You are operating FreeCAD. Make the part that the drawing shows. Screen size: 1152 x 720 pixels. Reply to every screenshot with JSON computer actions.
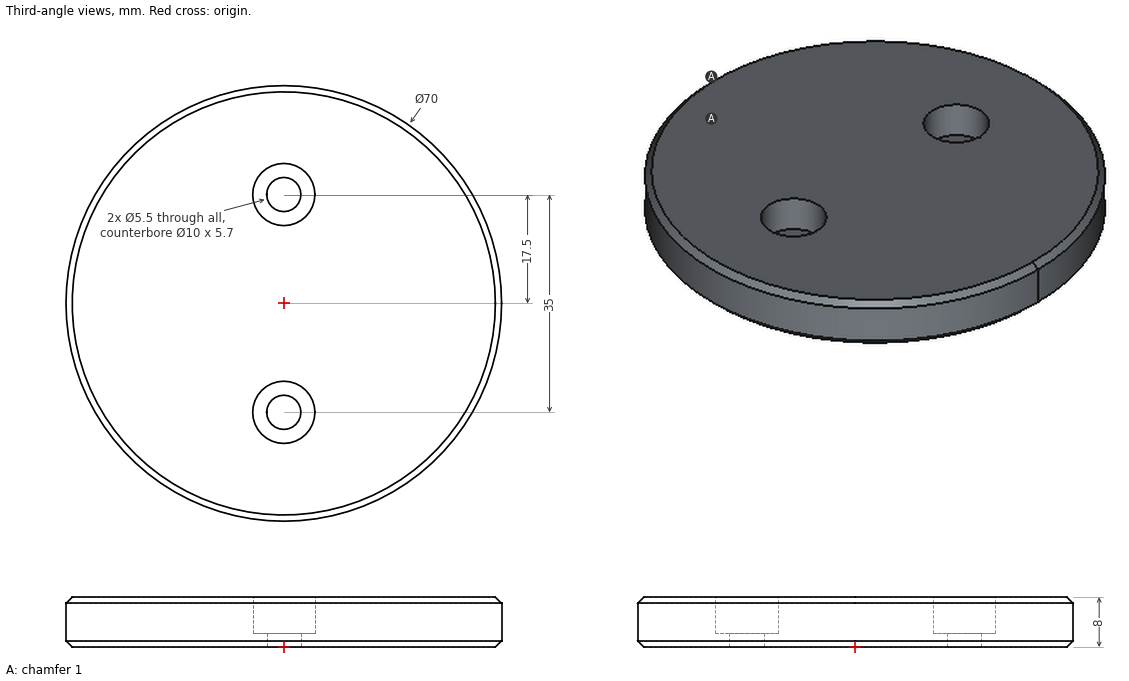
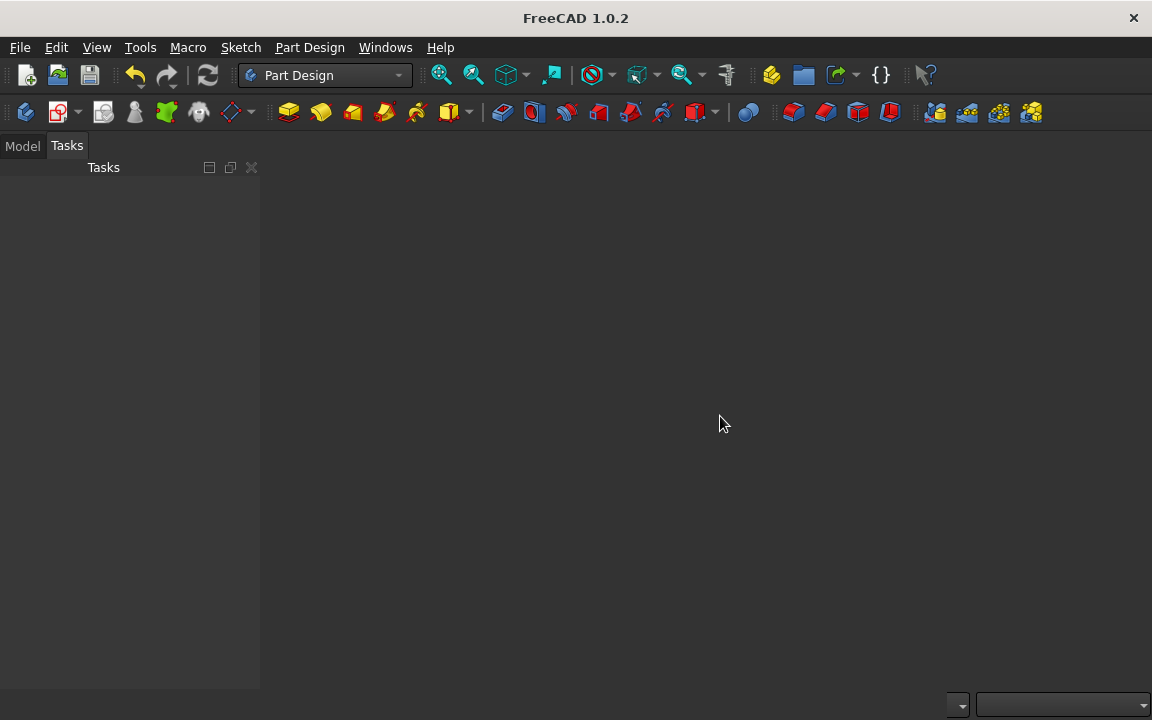
{"action": "key", "text": "ctrl+n"}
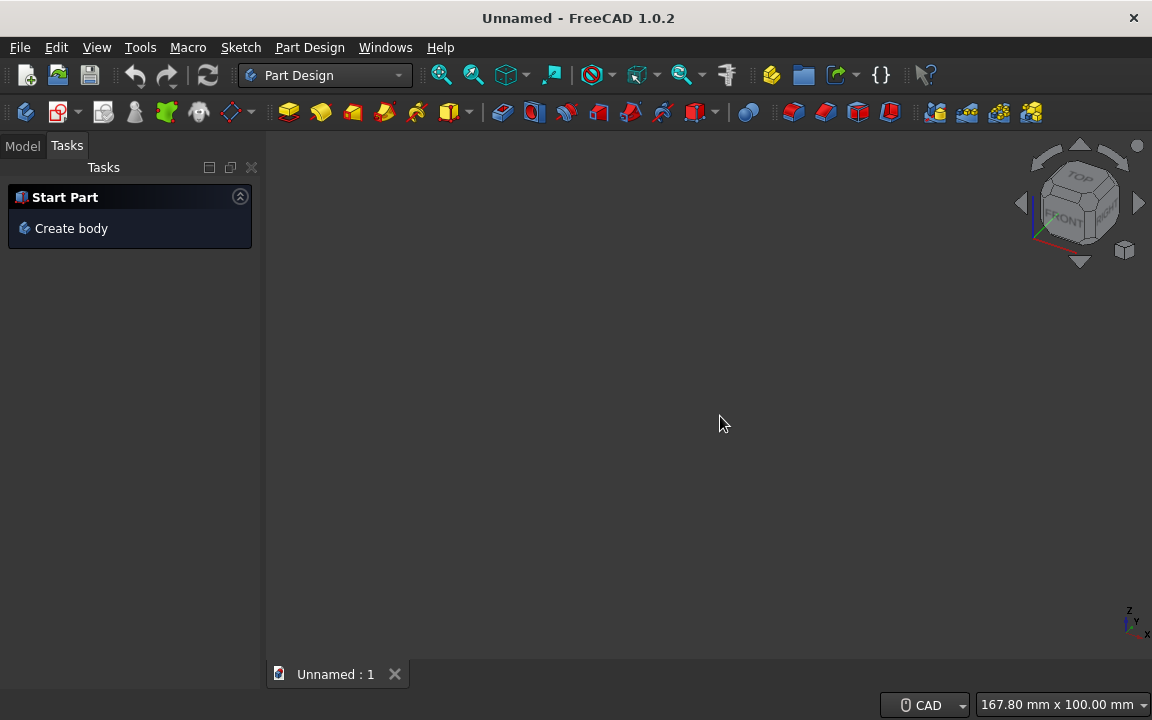
{"action": "left_click", "coordinate": [58, 112]}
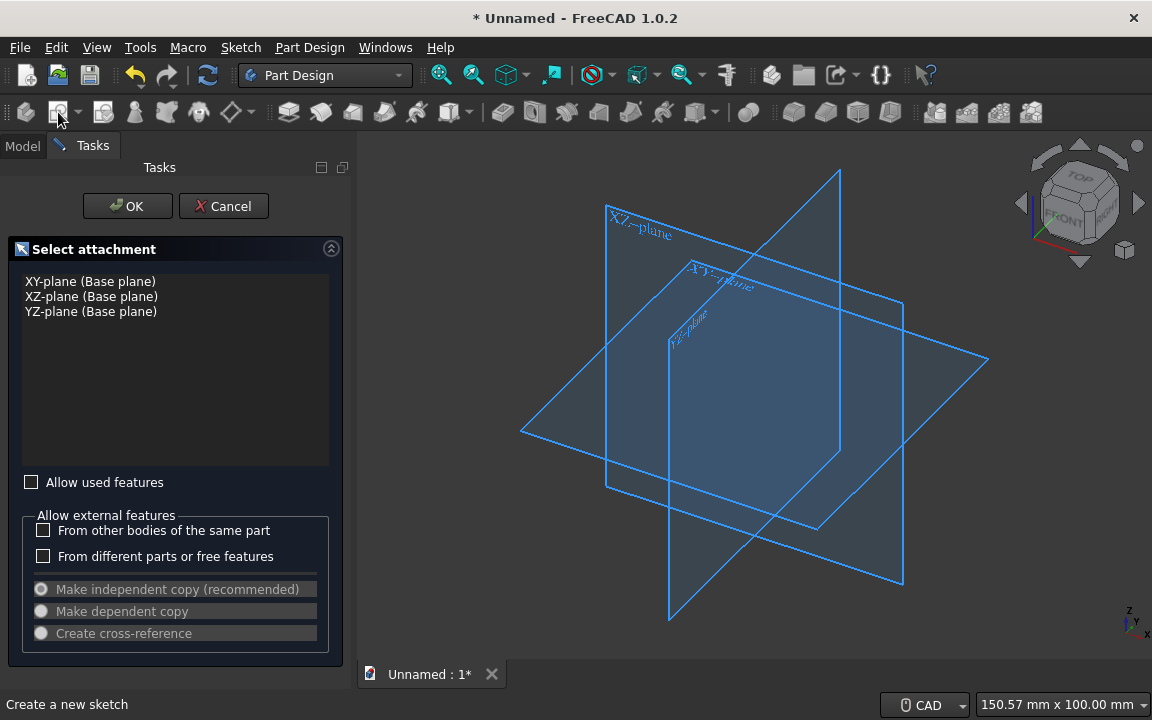
{"action": "left_click", "coordinate": [82, 282]}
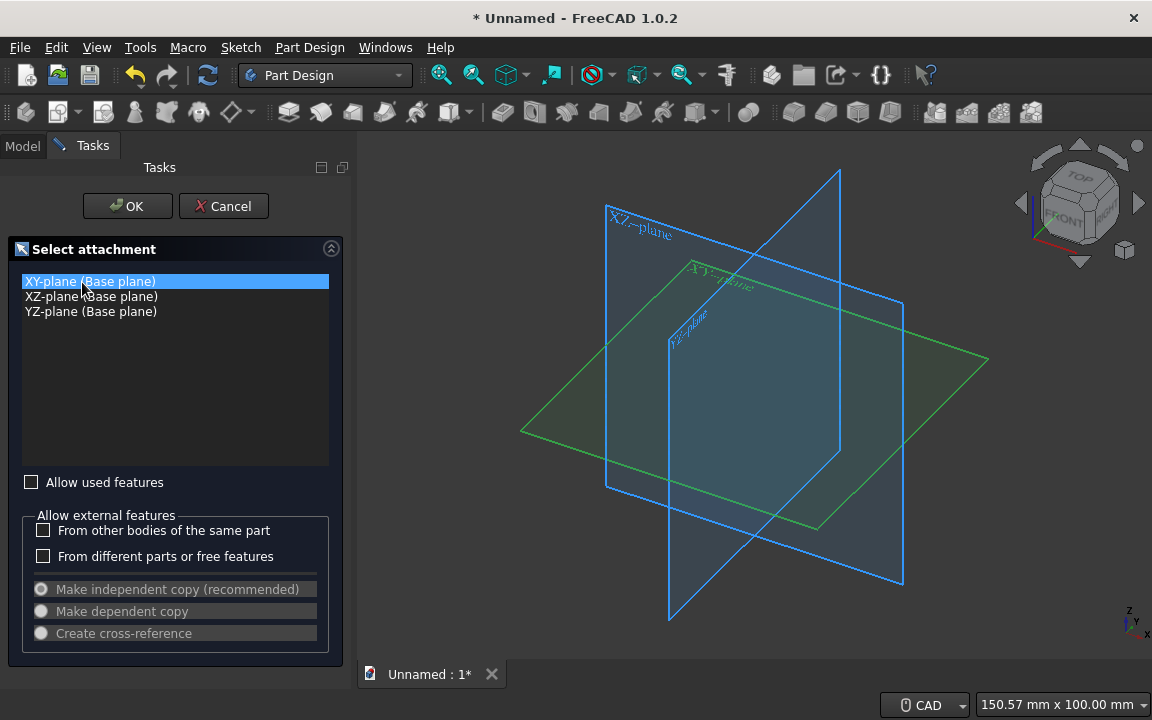
{"action": "left_click", "coordinate": [128, 206]}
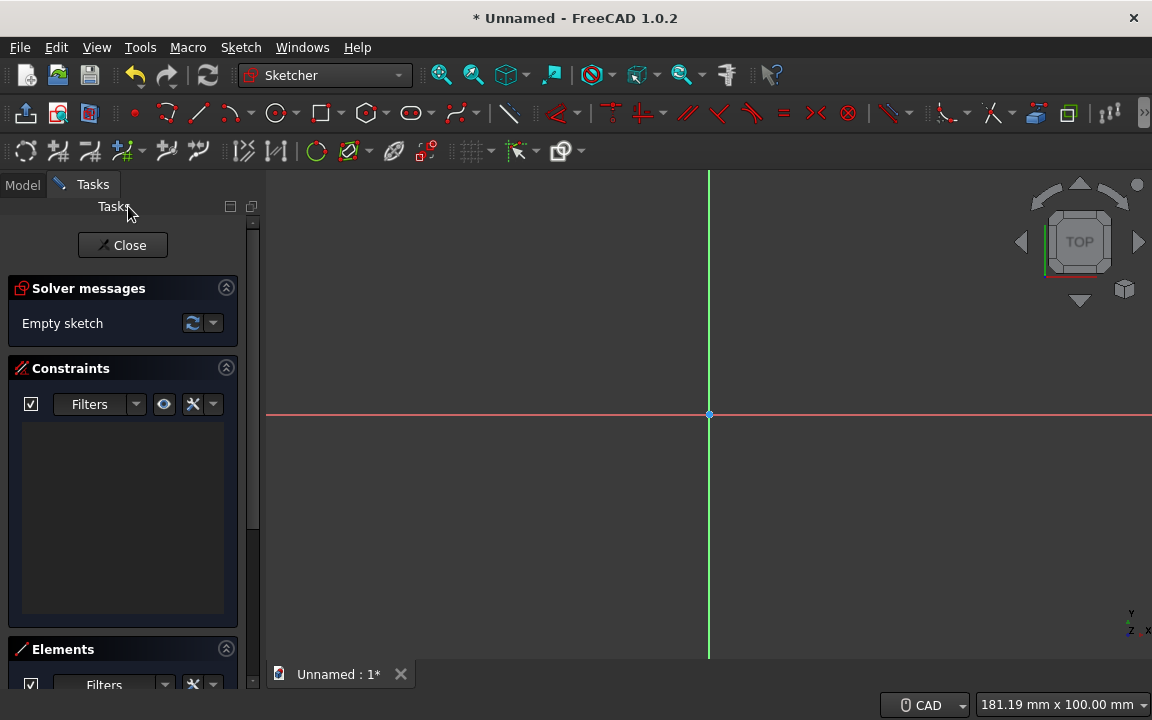
{"action": "left_click", "coordinate": [276, 114]}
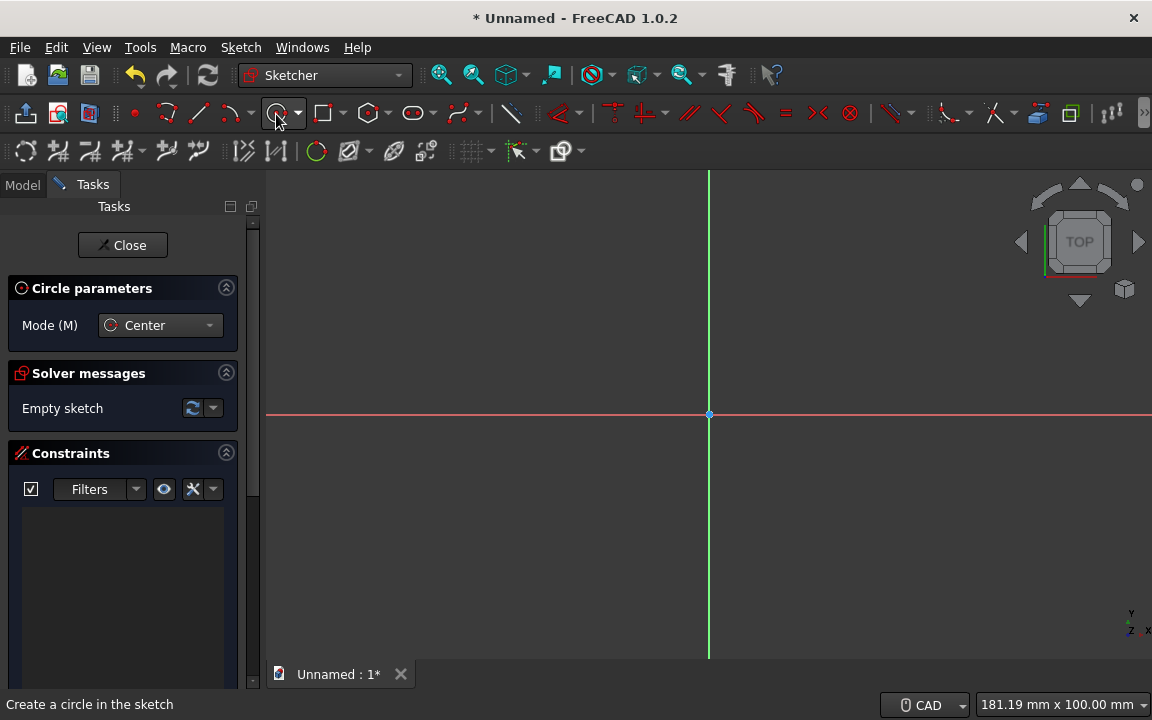
{"action": "left_click", "coordinate": [709, 414]}
{"action": "left_click", "coordinate": [830, 293]}
{"action": "key", "text": "Escape"}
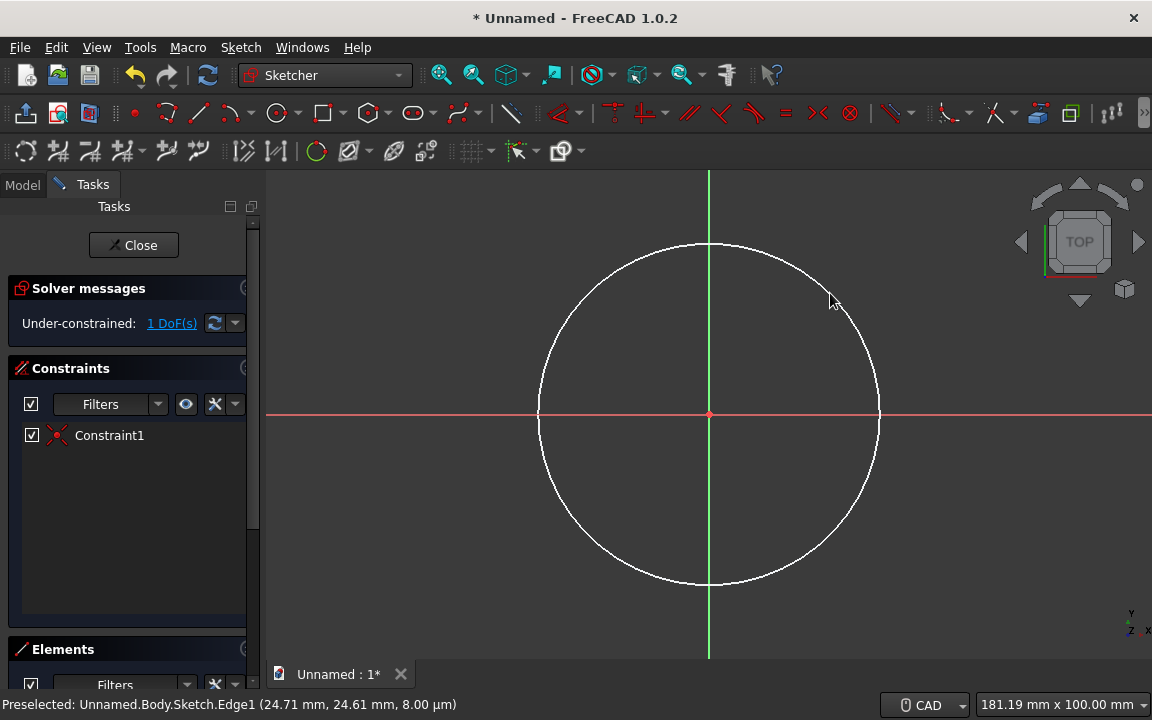
{"action": "left_click", "coordinate": [558, 114]}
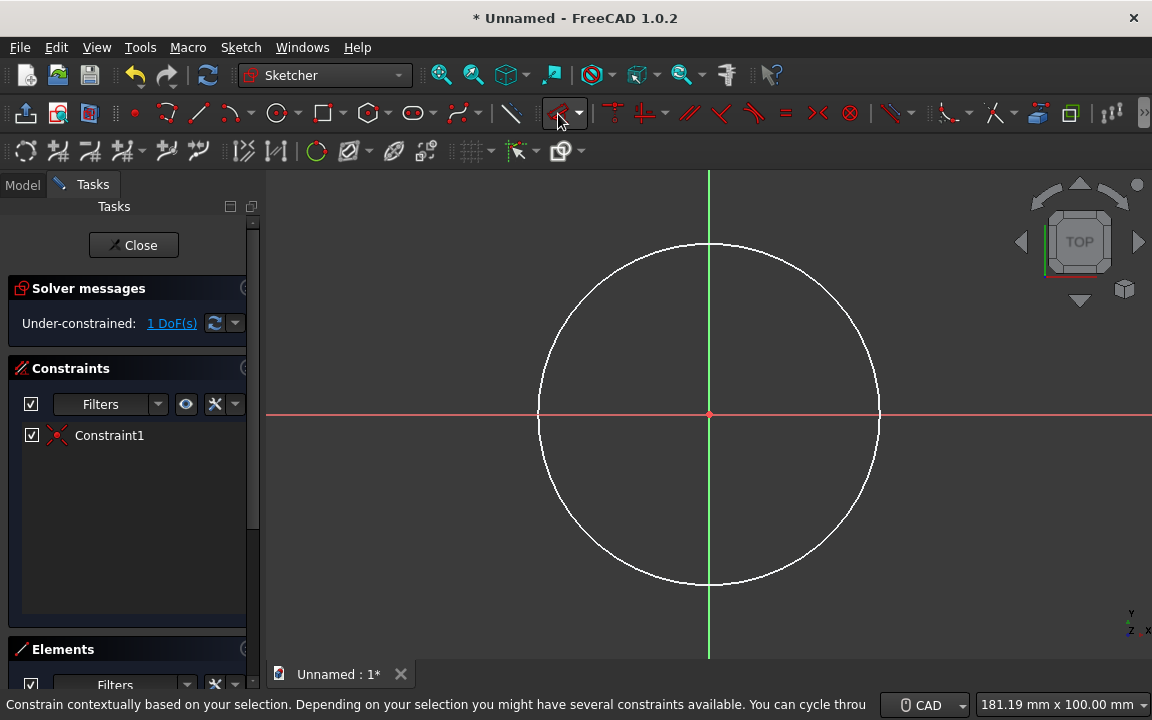
{"action": "left_click", "coordinate": [829, 293]}
{"action": "left_click", "coordinate": [851, 270]}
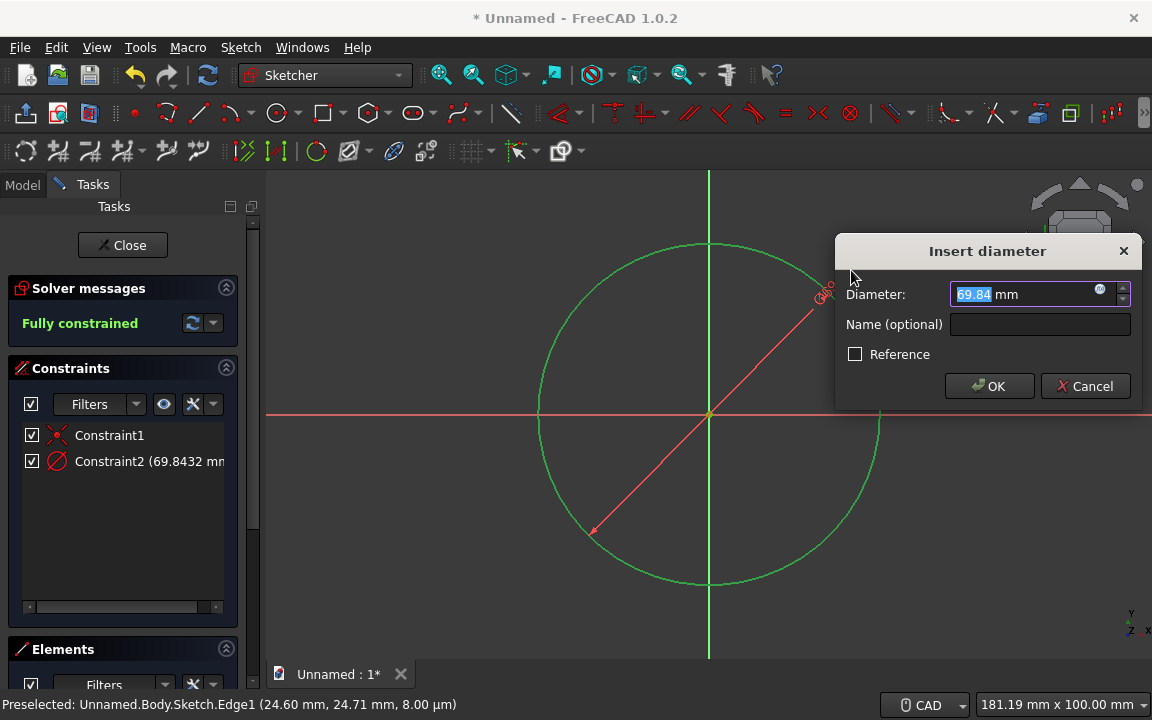
{"action": "type", "text": "70"}
{"action": "key", "text": "Return"}
{"action": "key", "text": "Escape"}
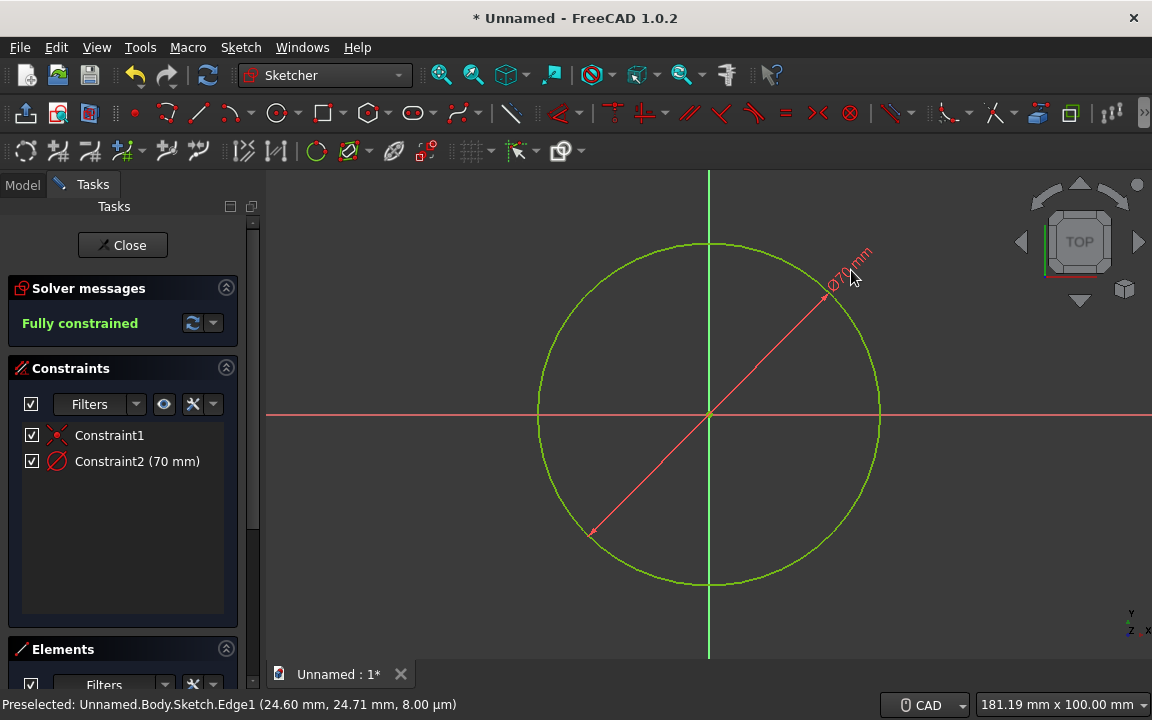
{"action": "left_click", "coordinate": [123, 245]}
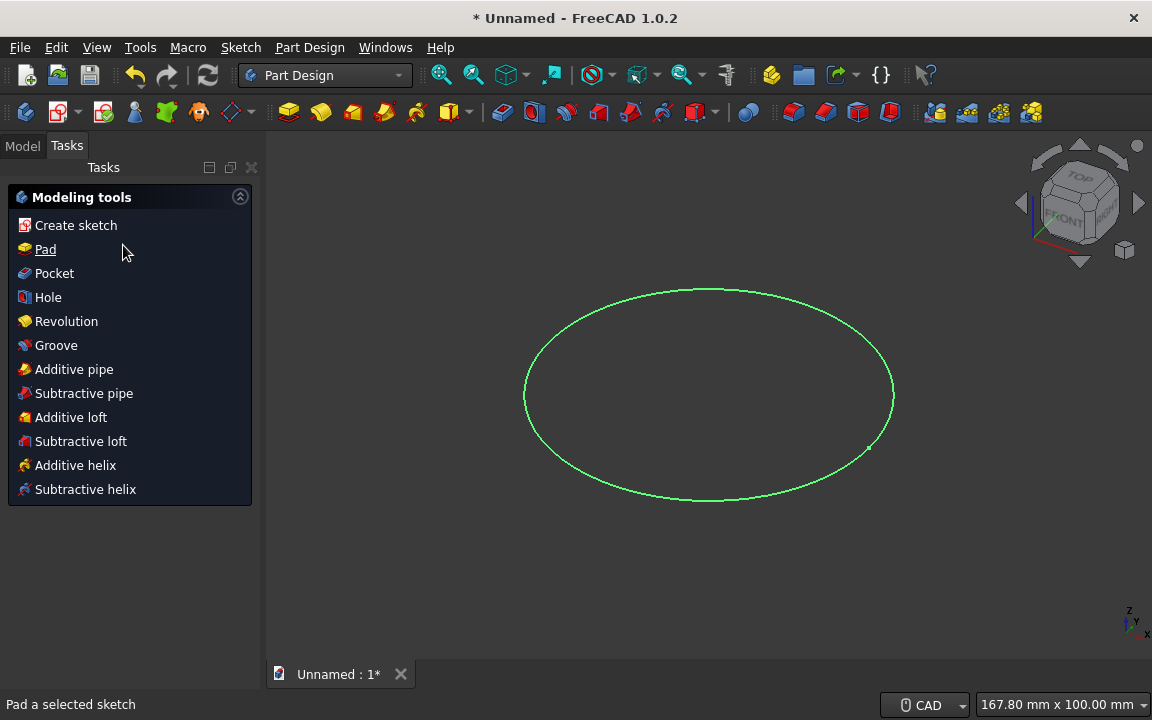
{"action": "left_click", "coordinate": [290, 112]}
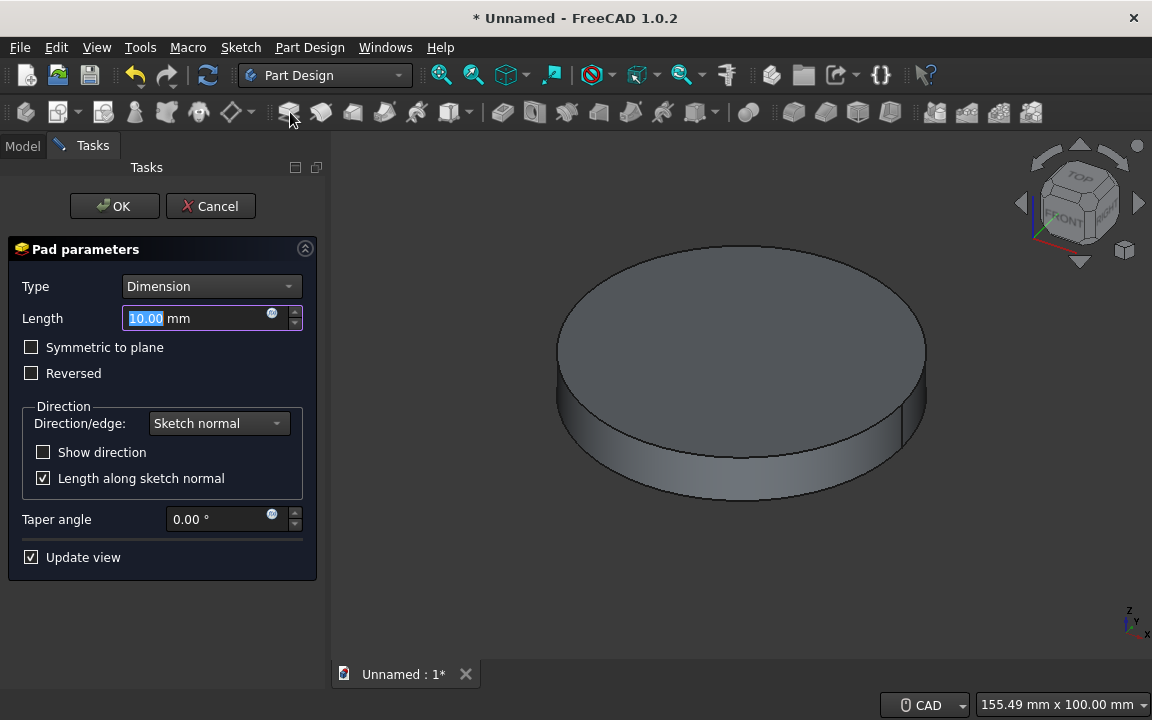
{"action": "type", "text": "8"}
{"action": "key", "text": "Tab"}